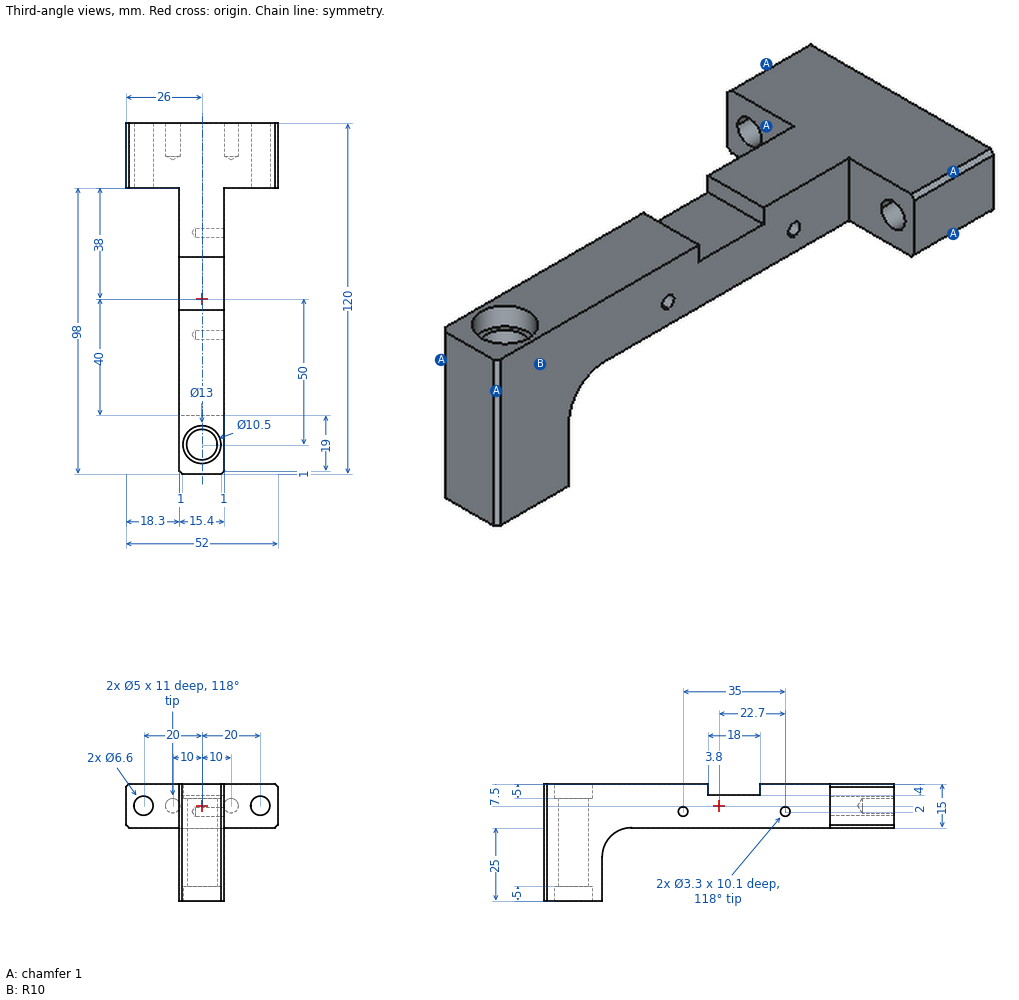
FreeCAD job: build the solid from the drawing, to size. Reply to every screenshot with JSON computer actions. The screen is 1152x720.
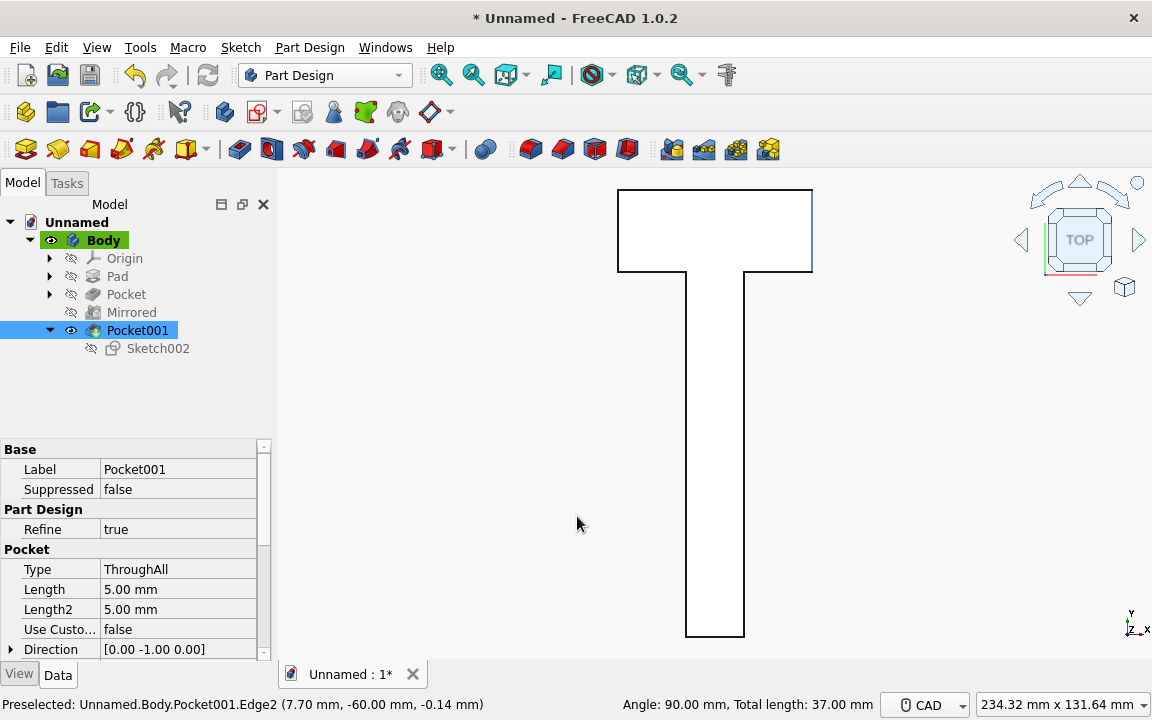
{"action": "left_click", "coordinate": [618, 230], "text": "ctrl"}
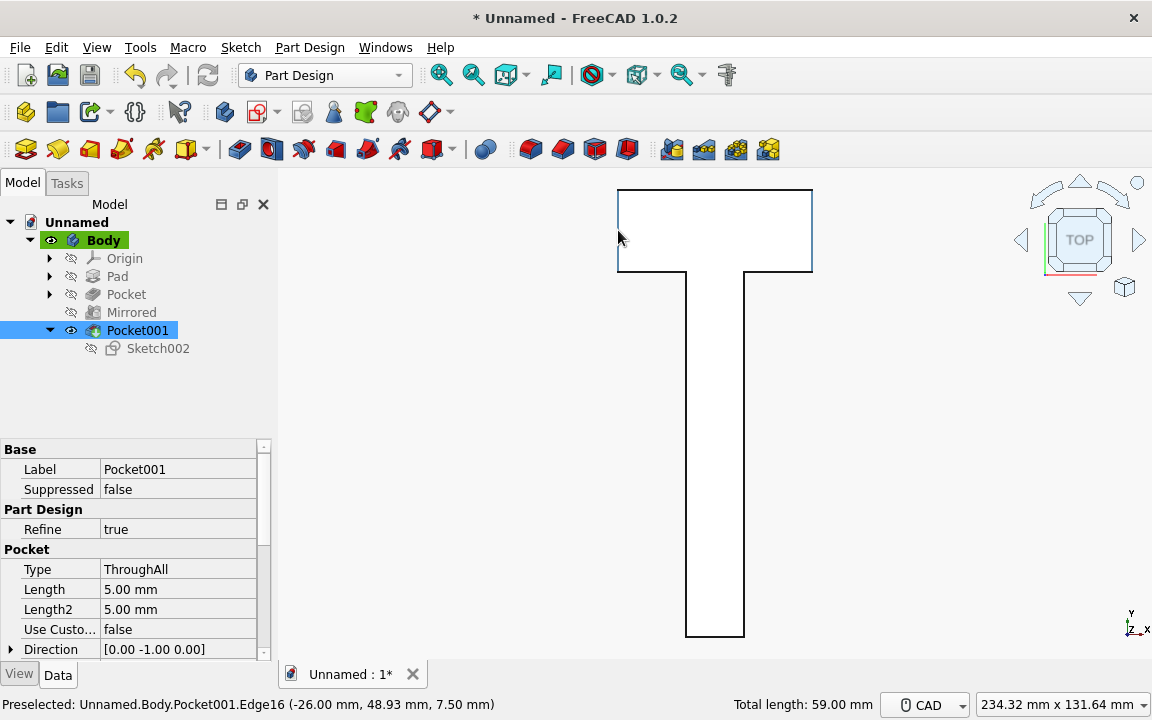
{"action": "key", "text": "1"}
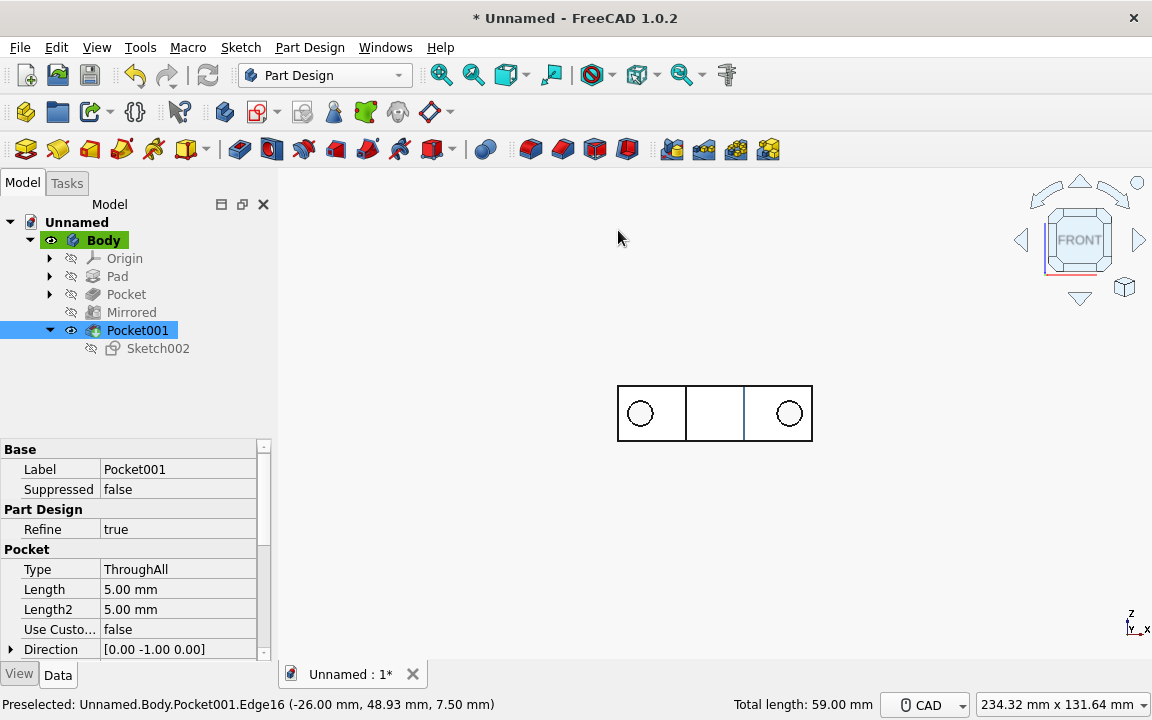
{"action": "left_click", "coordinate": [442, 76]}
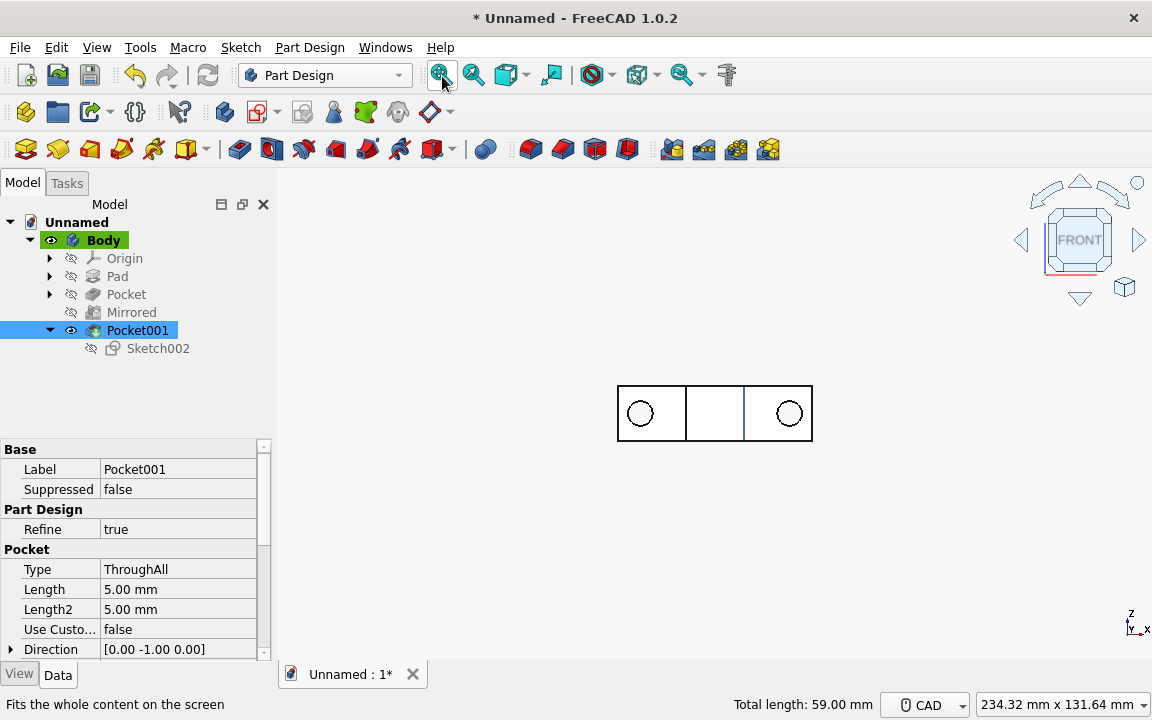
{"action": "left_click", "coordinate": [686, 413], "text": "ctrl"}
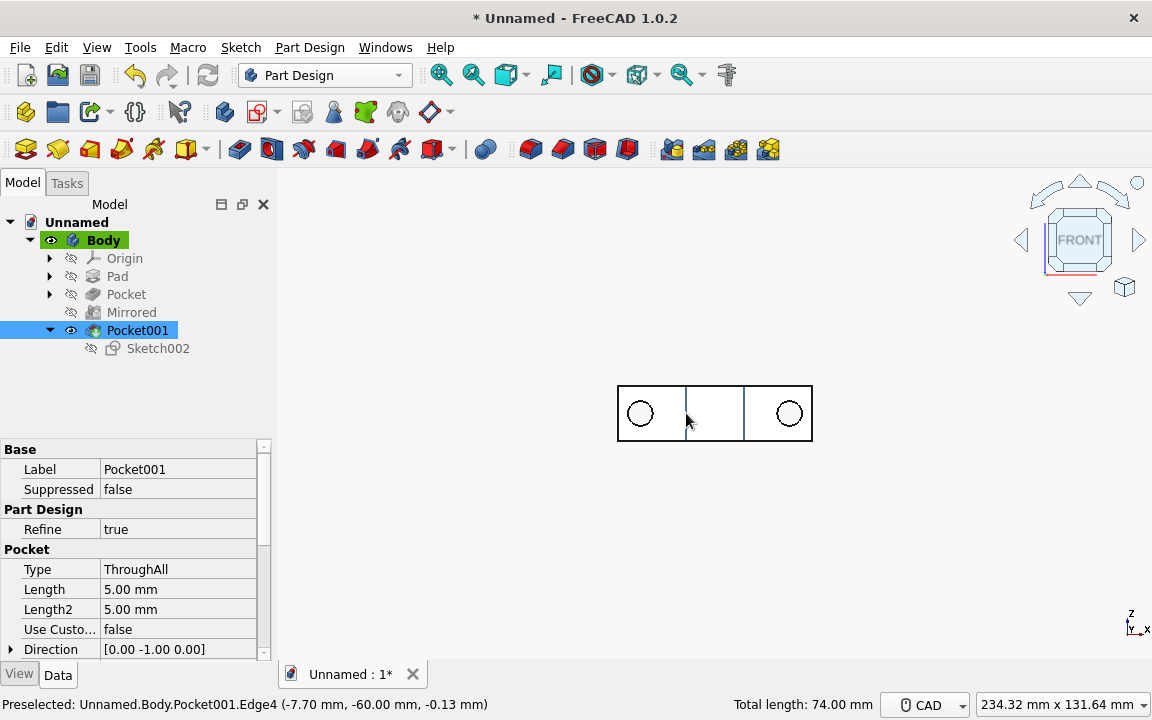
{"action": "key", "text": "3"}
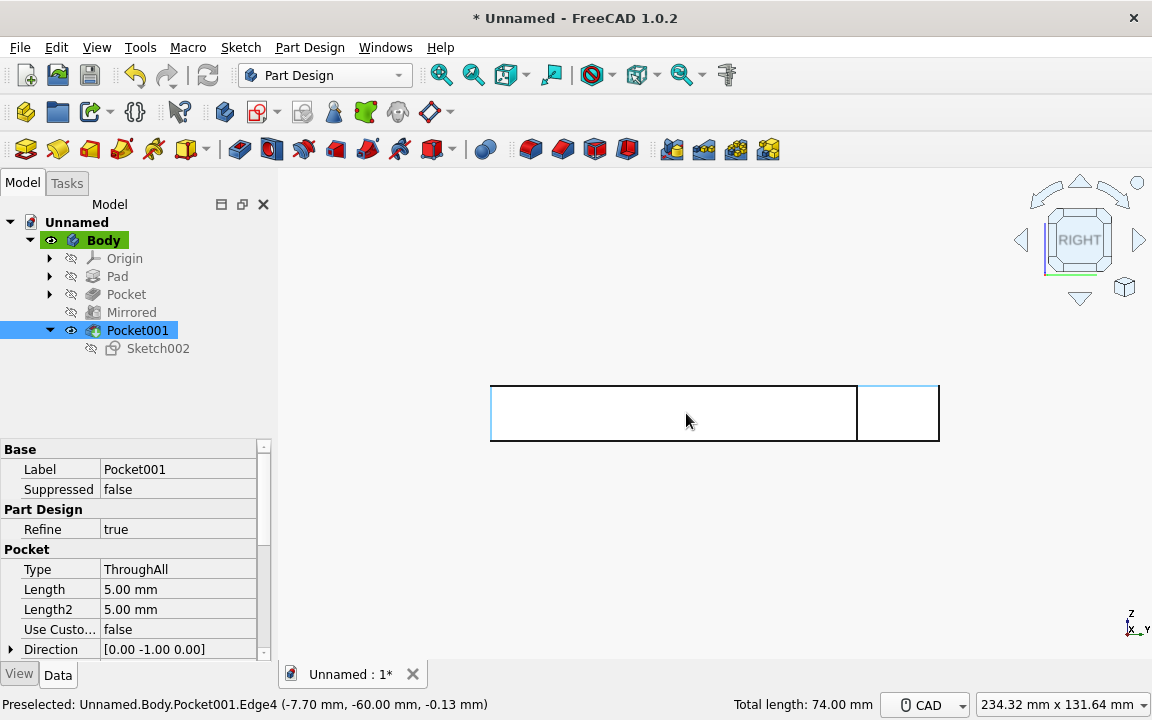
{"action": "left_click", "coordinate": [898, 440], "text": "ctrl"}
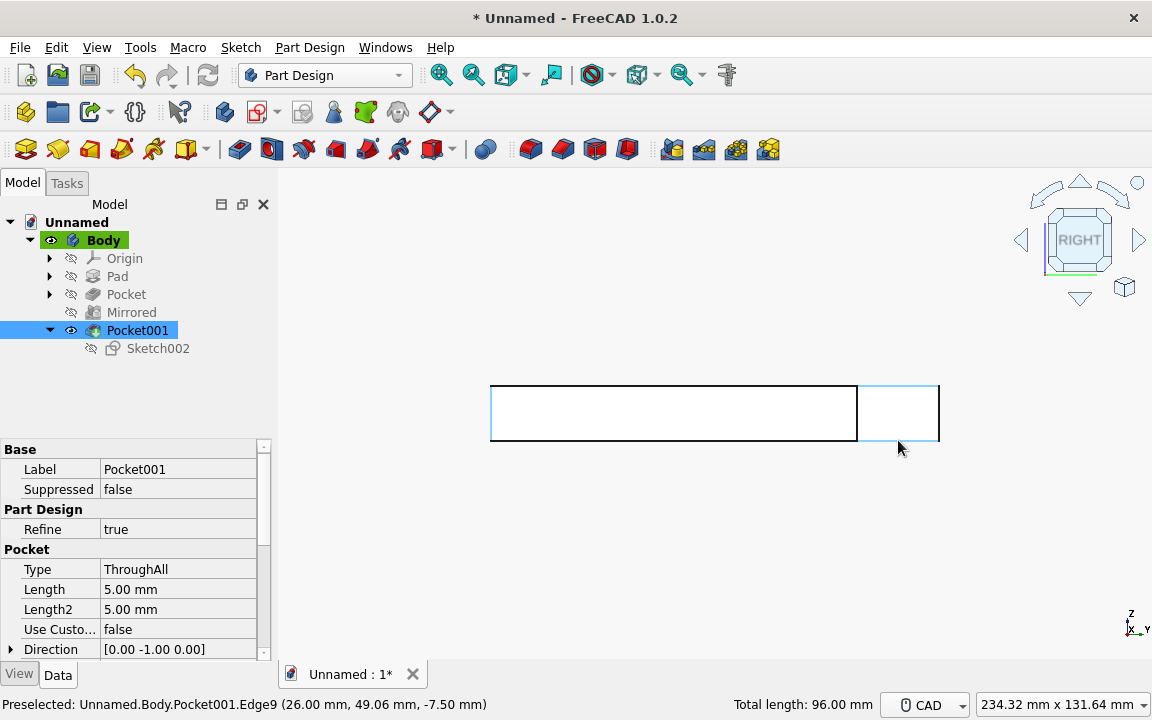
{"action": "key", "text": "5"}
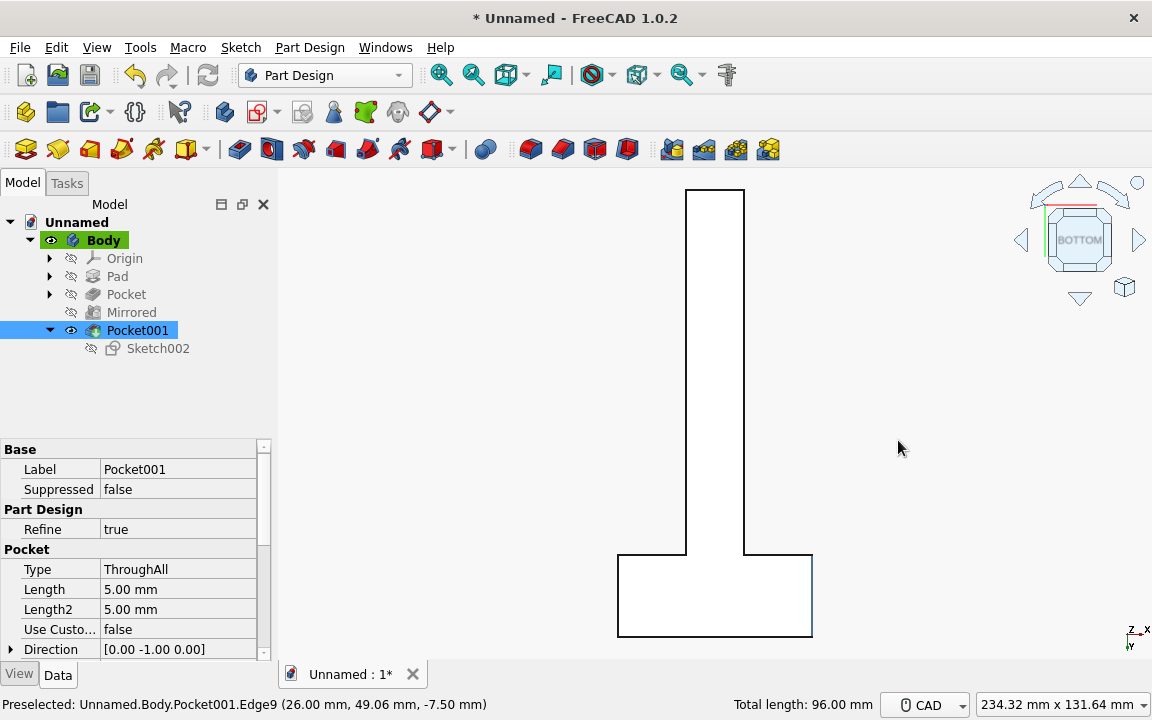
{"action": "left_click", "coordinate": [618, 595], "text": "ctrl"}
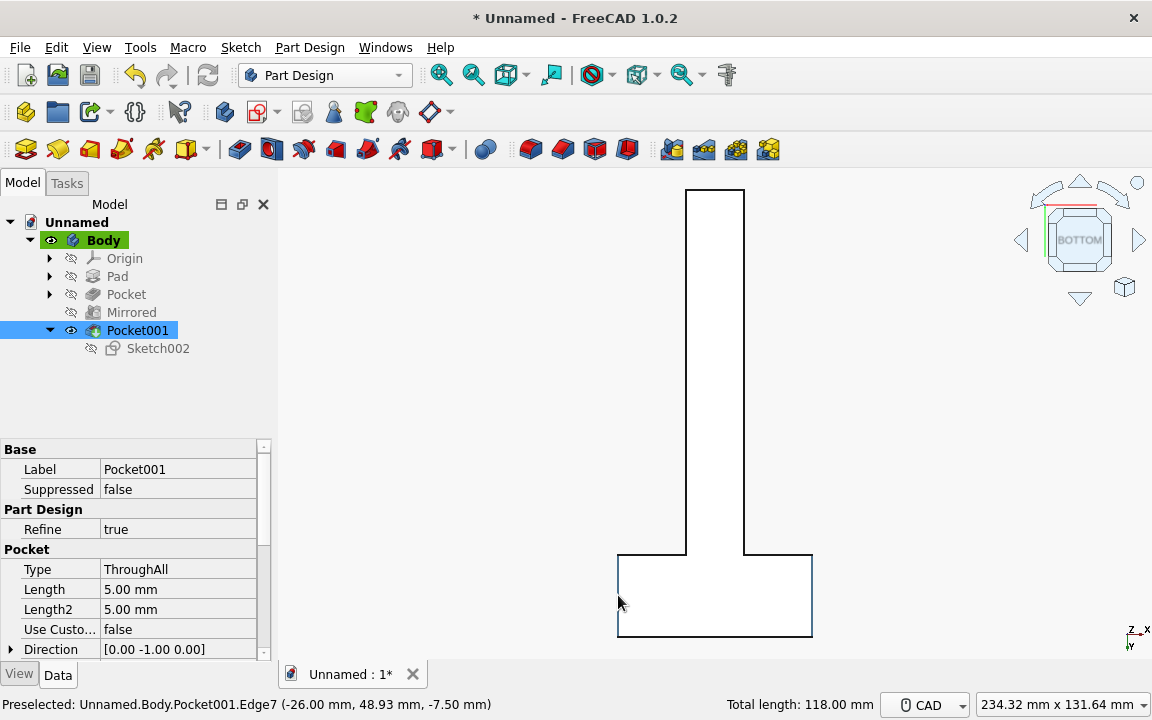
{"action": "left_click", "coordinate": [564, 150]}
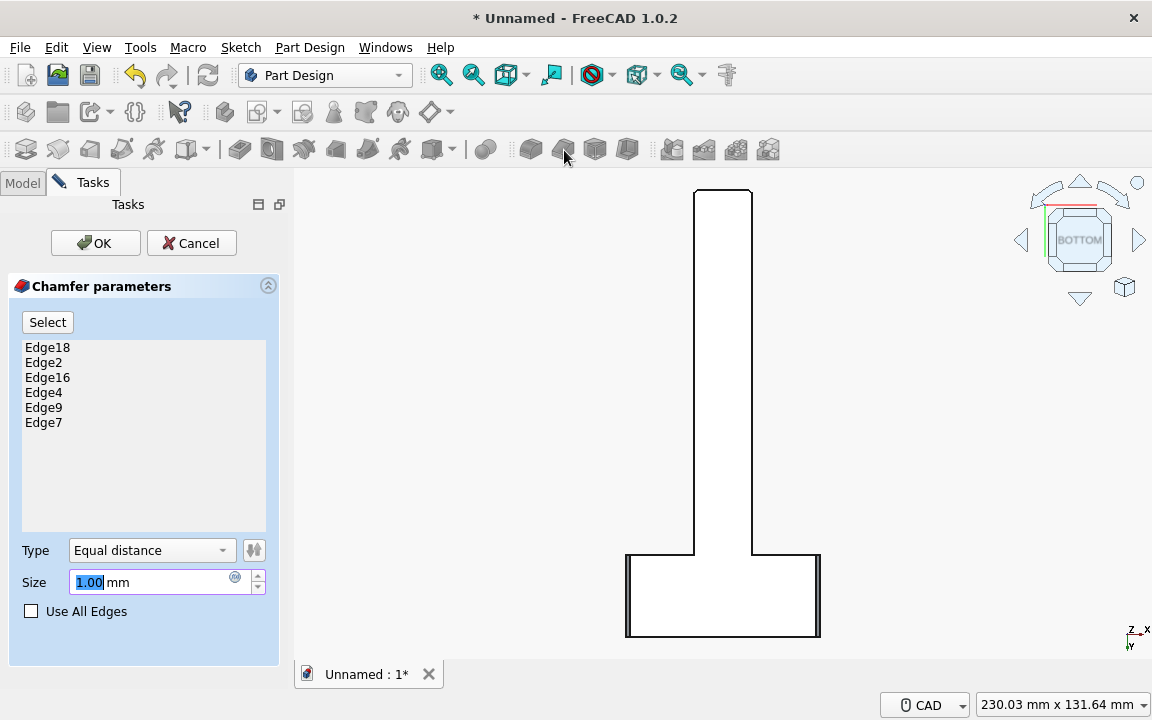
{"action": "type", "text": "1"}
{"action": "key", "text": "Tab"}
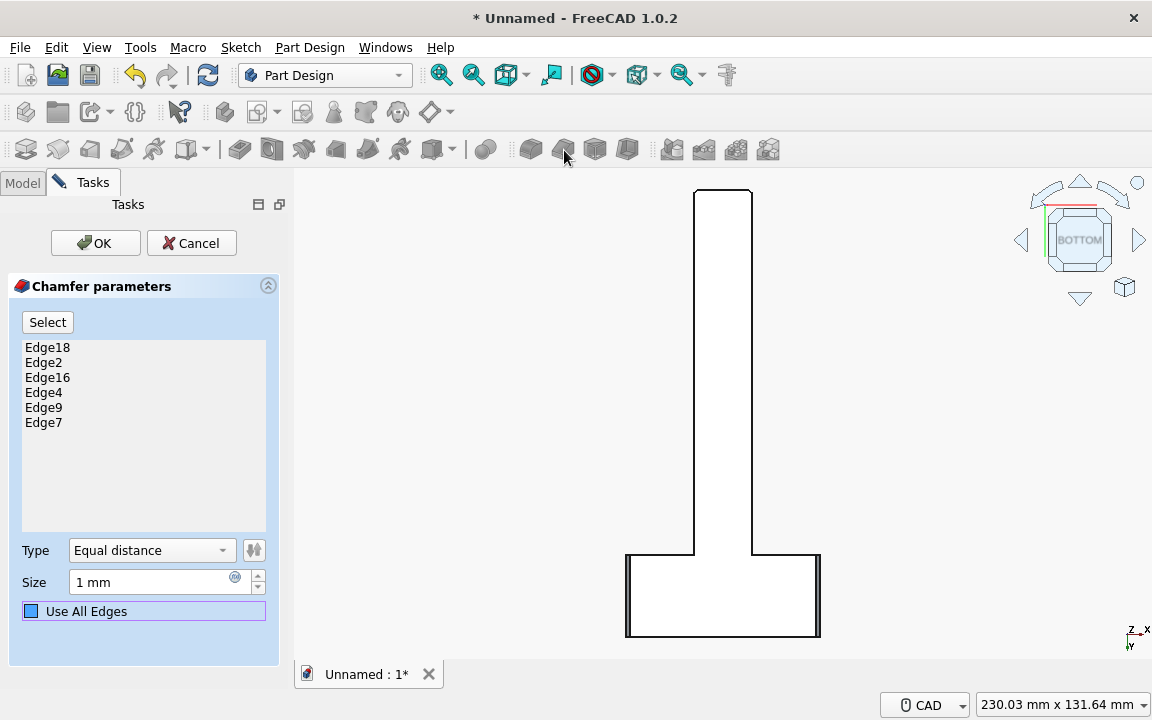
{"action": "left_click", "coordinate": [96, 243]}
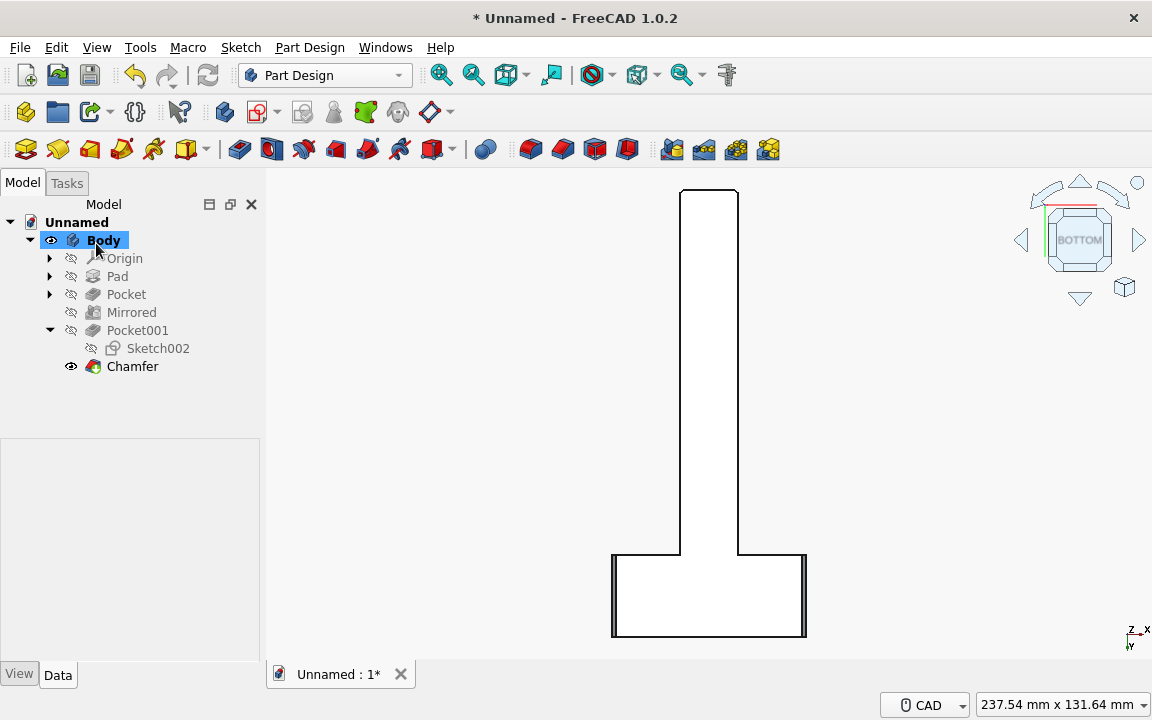
{"action": "key", "text": "4"}